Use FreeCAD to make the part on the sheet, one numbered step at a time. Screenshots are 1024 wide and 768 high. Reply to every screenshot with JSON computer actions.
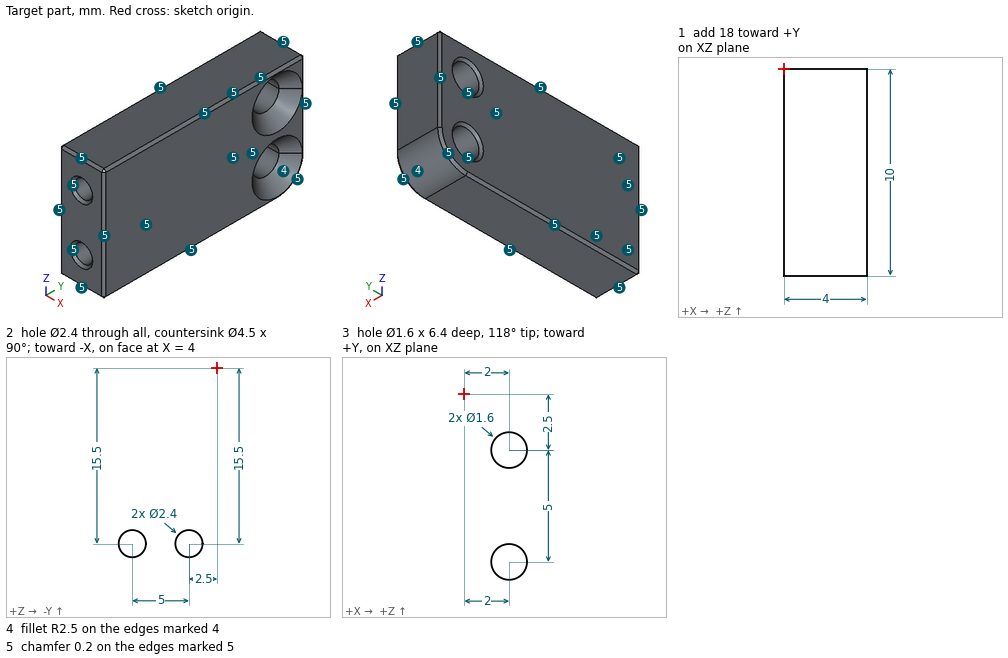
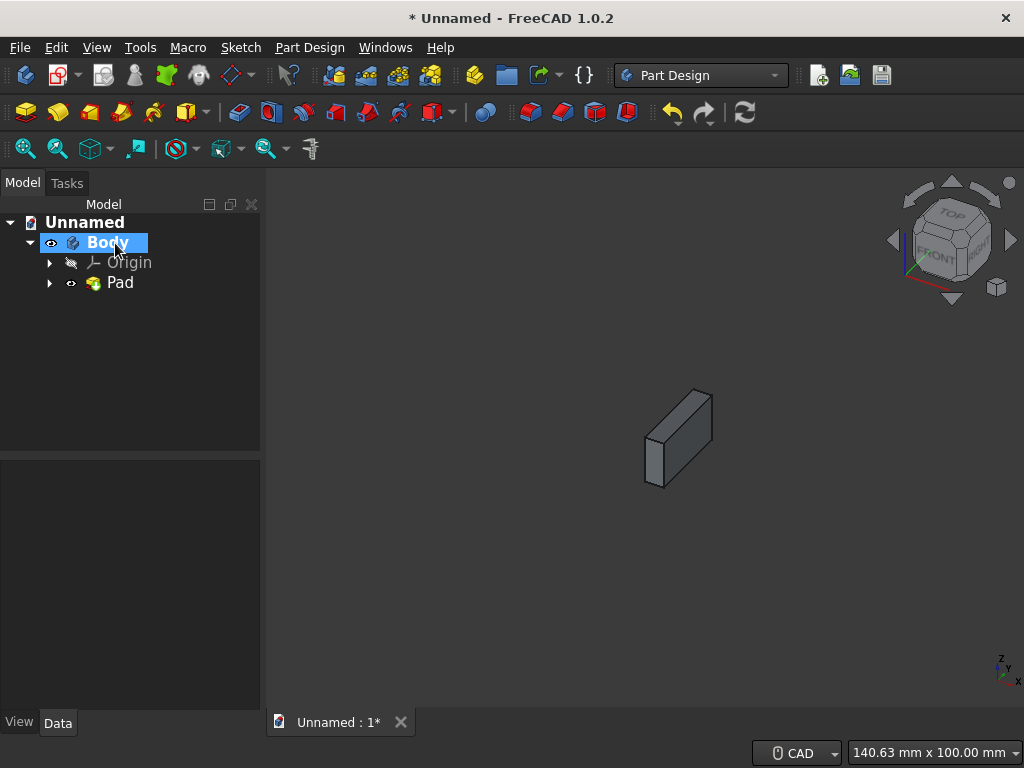
{"action": "left_click", "coordinate": [26, 150]}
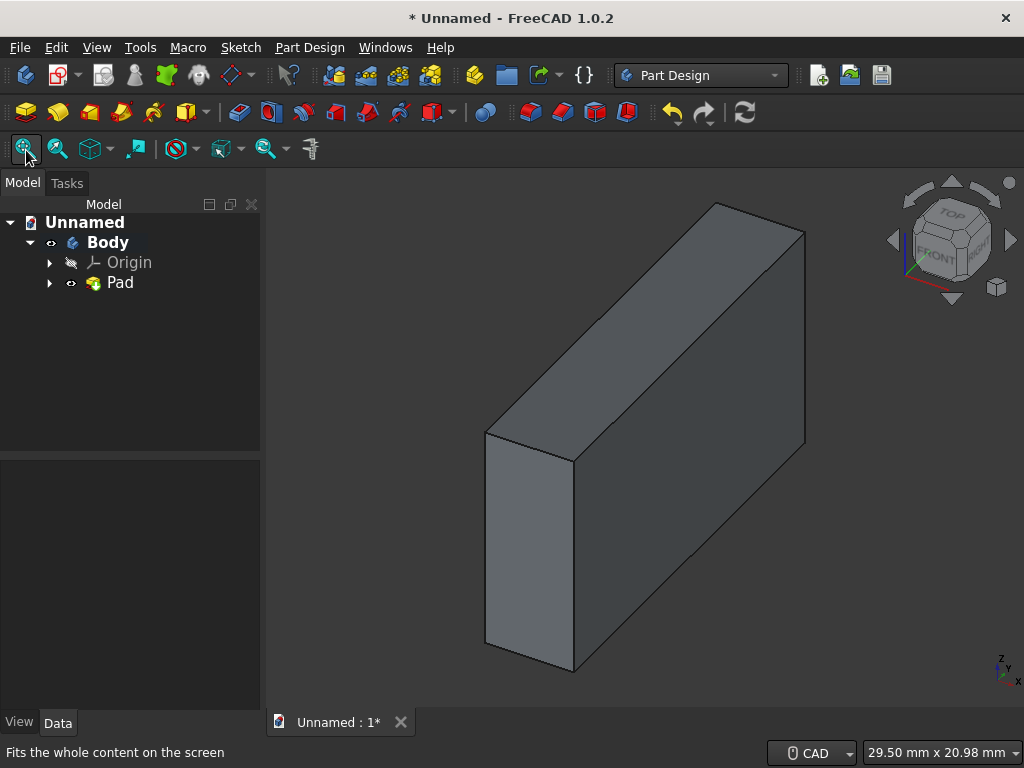
{"action": "left_click", "coordinate": [690, 451]}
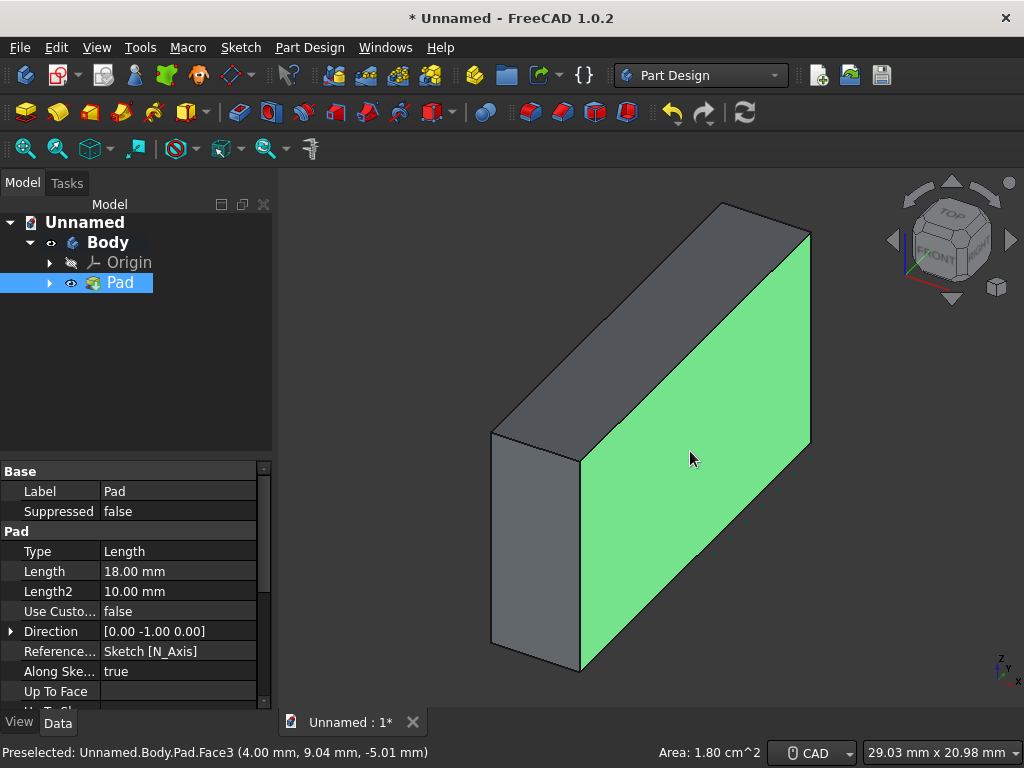
{"action": "left_click", "coordinate": [58, 76]}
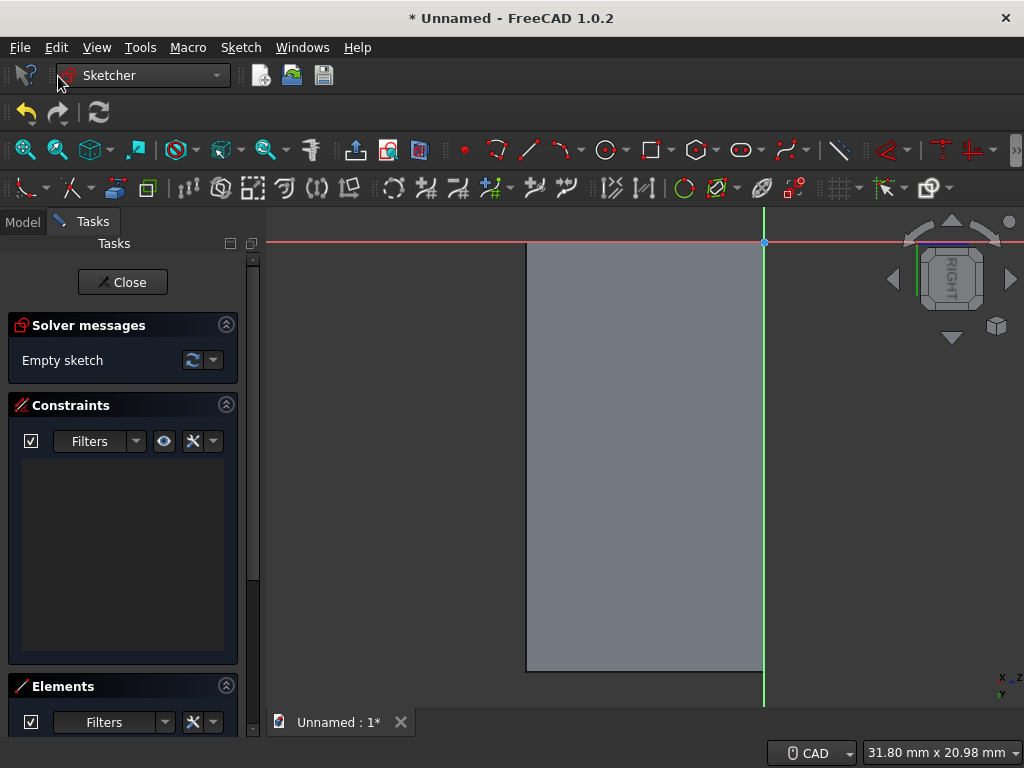
{"action": "scroll", "coordinate": [294, 527], "scroll_direction": "down", "scroll_amount": 1}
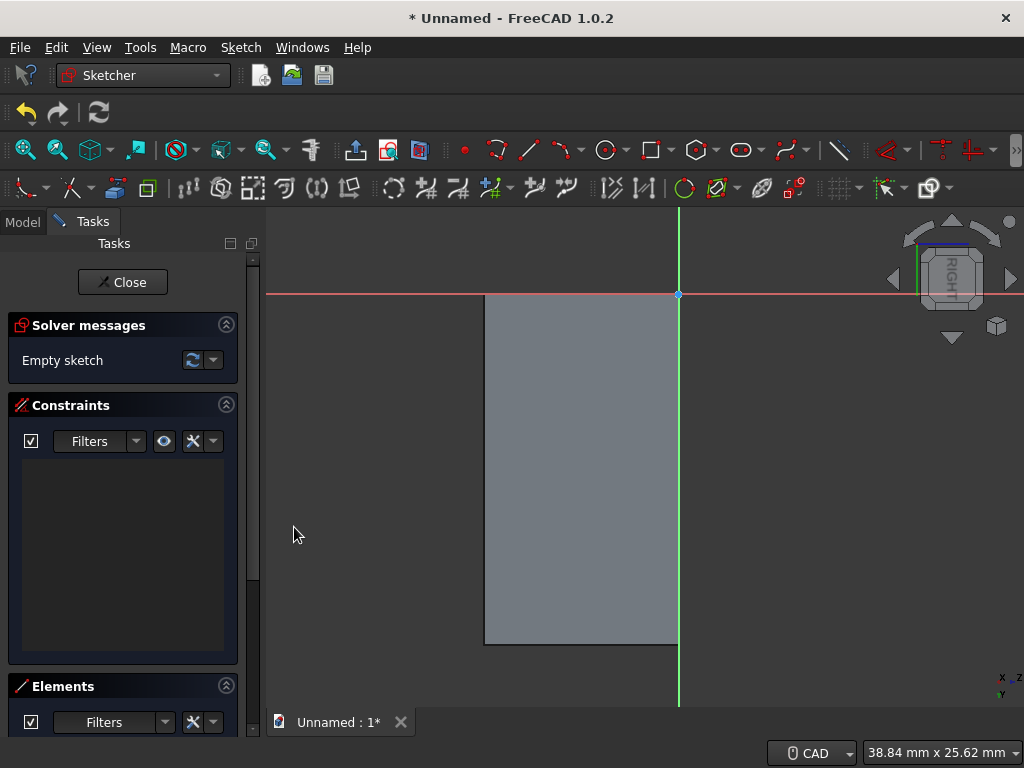
{"action": "key", "text": "g c"}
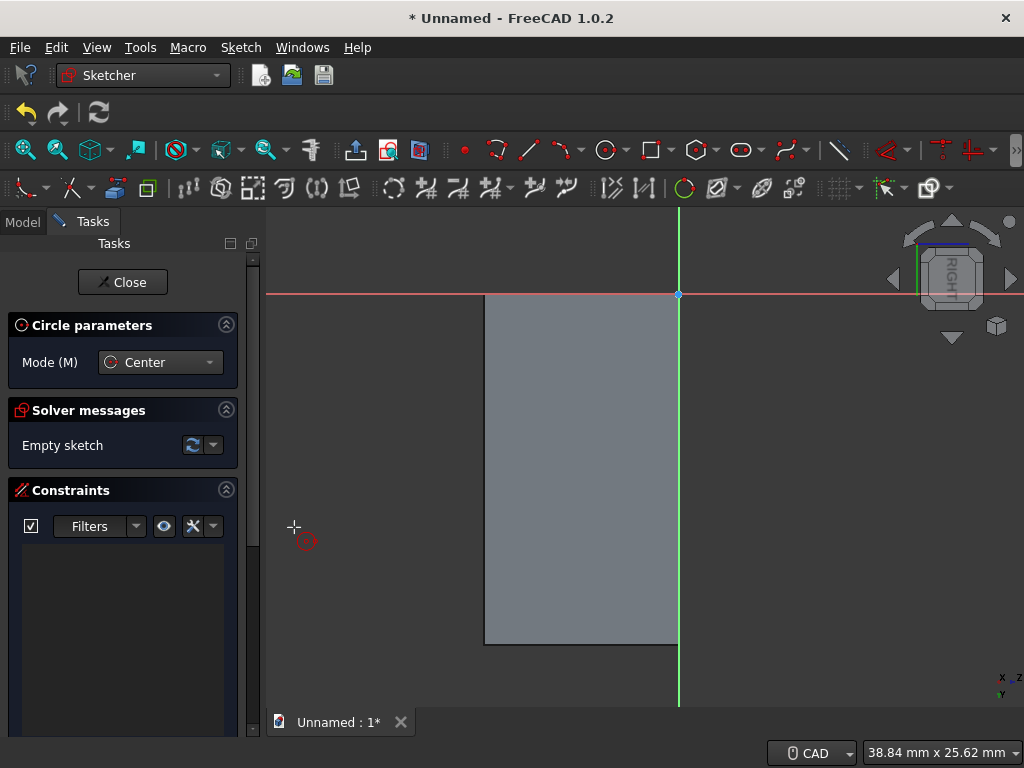
{"action": "left_click", "coordinate": [630, 597]}
{"action": "mouse_move", "coordinate": [647, 580]}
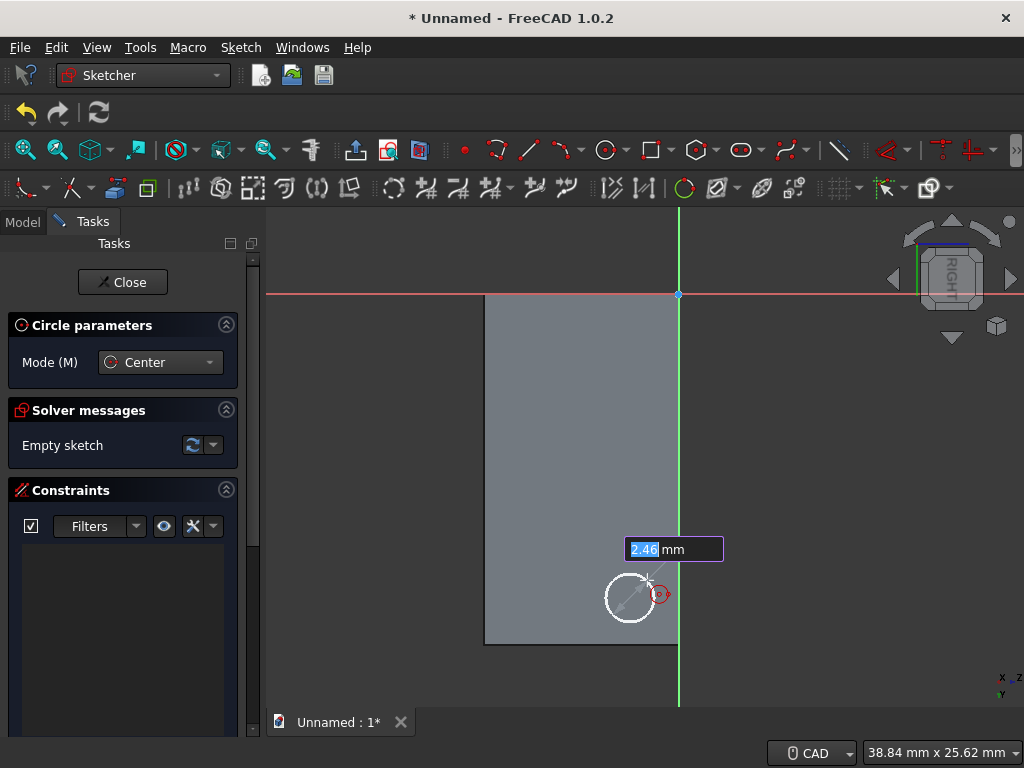
{"action": "type", "text": "2.4"}
{"action": "key", "text": "Return"}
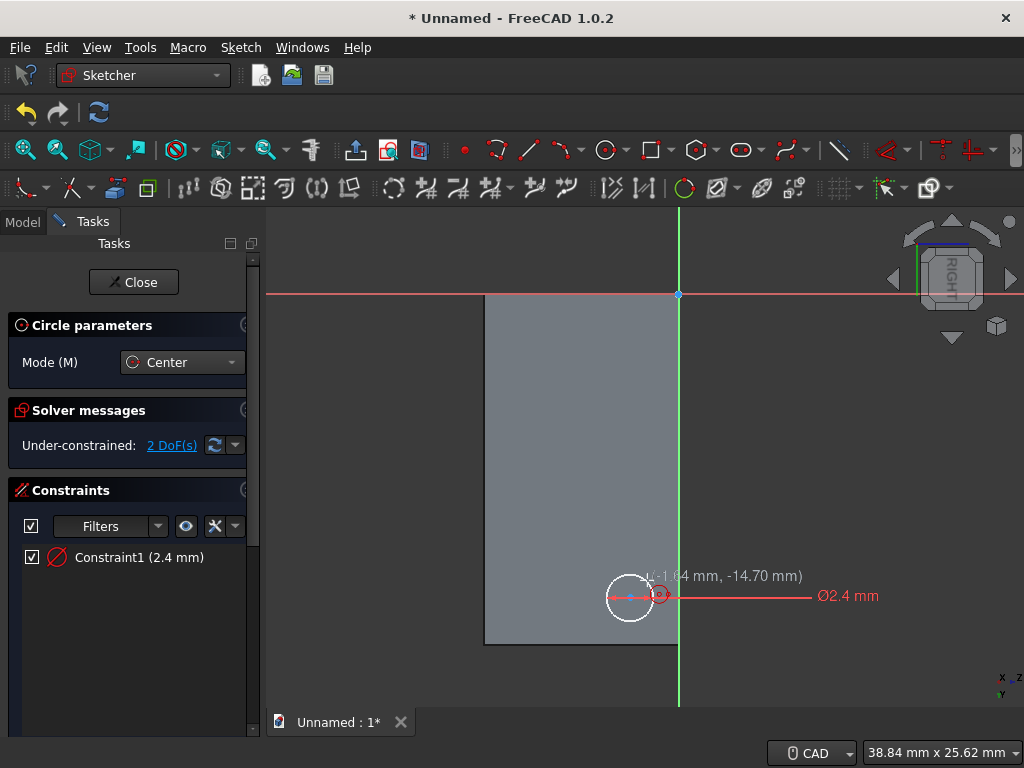
{"action": "left_click", "coordinate": [533, 597]}
{"action": "mouse_move", "coordinate": [549, 580]}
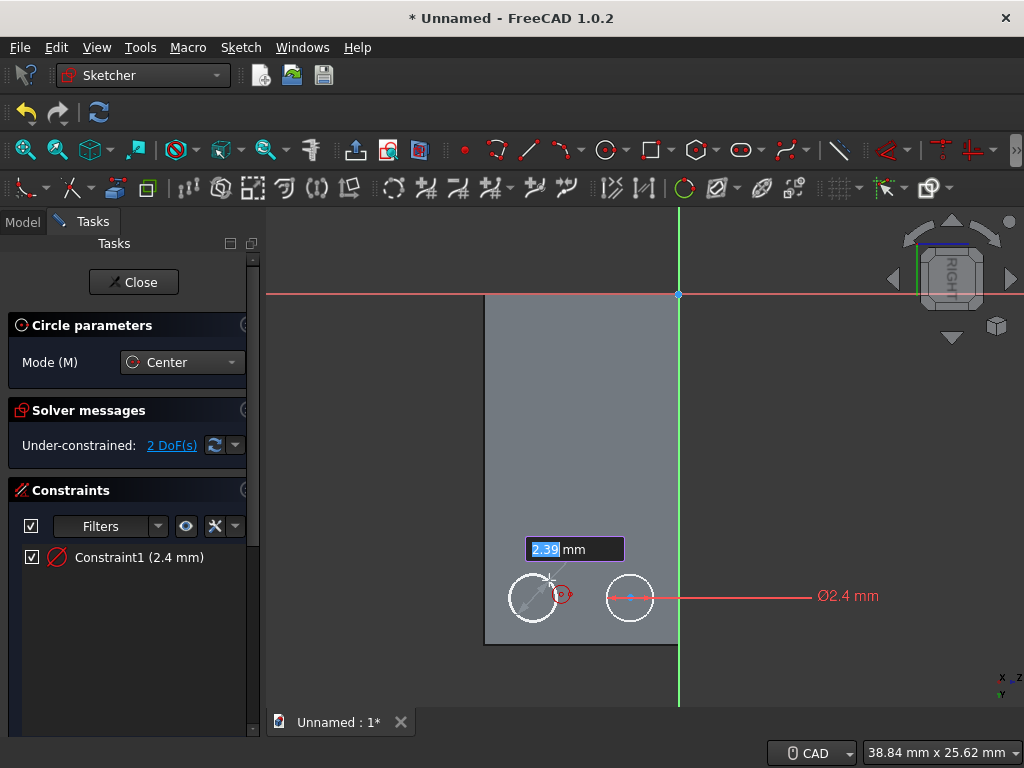
{"action": "type", "text": "2.4"}
{"action": "key", "text": "Return"}
{"action": "key", "text": "Escape"}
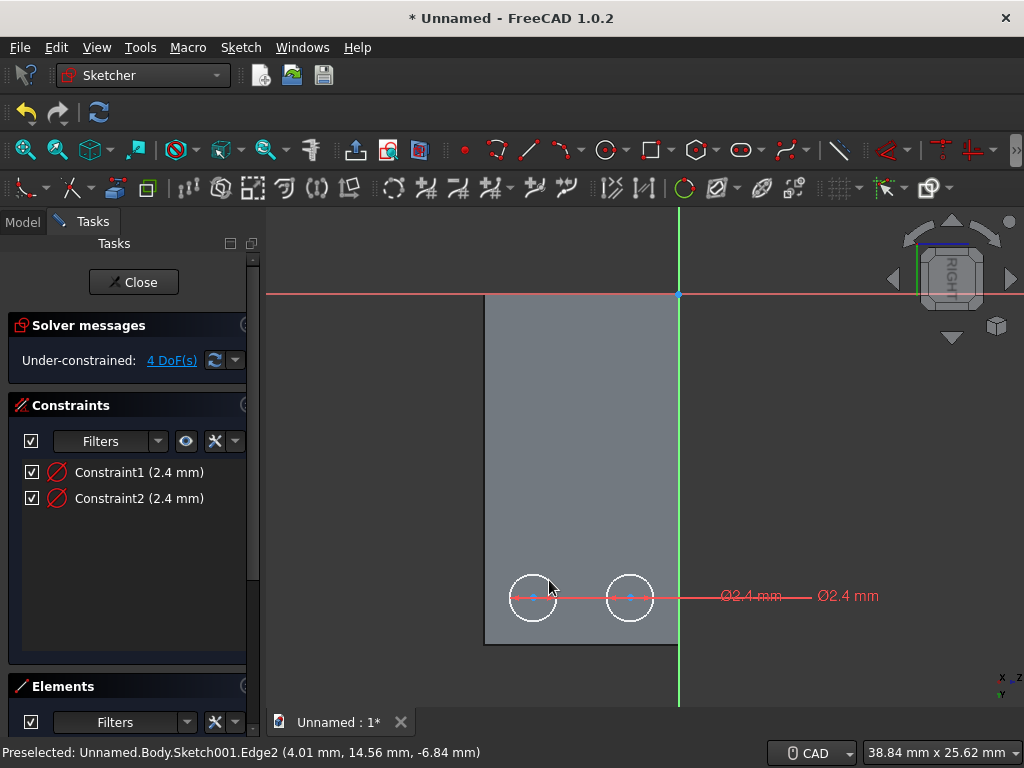
{"action": "key", "text": "d"}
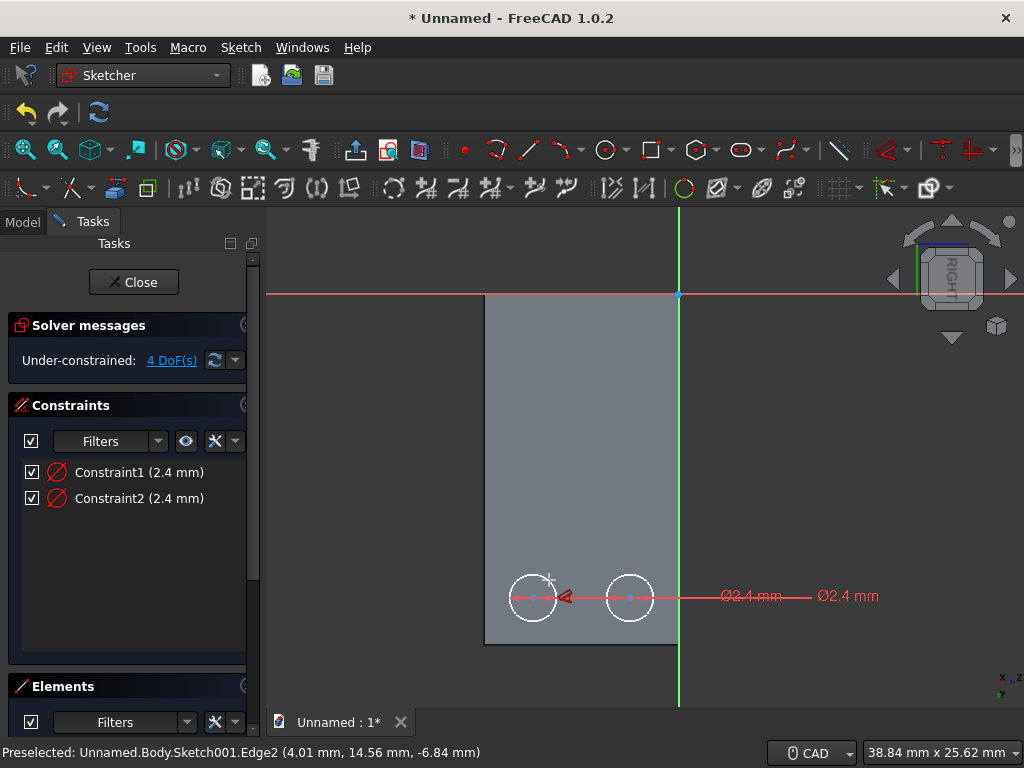
{"action": "left_click", "coordinate": [630, 598]}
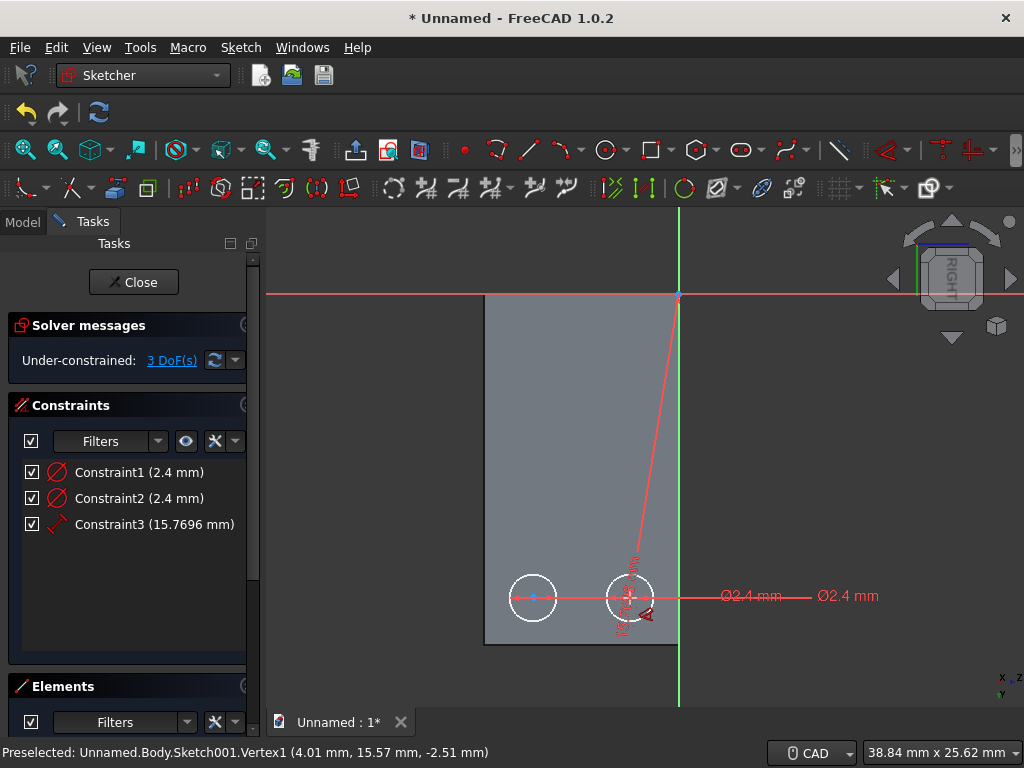
{"action": "left_click", "coordinate": [533, 598]}
{"action": "left_click", "coordinate": [581, 632]}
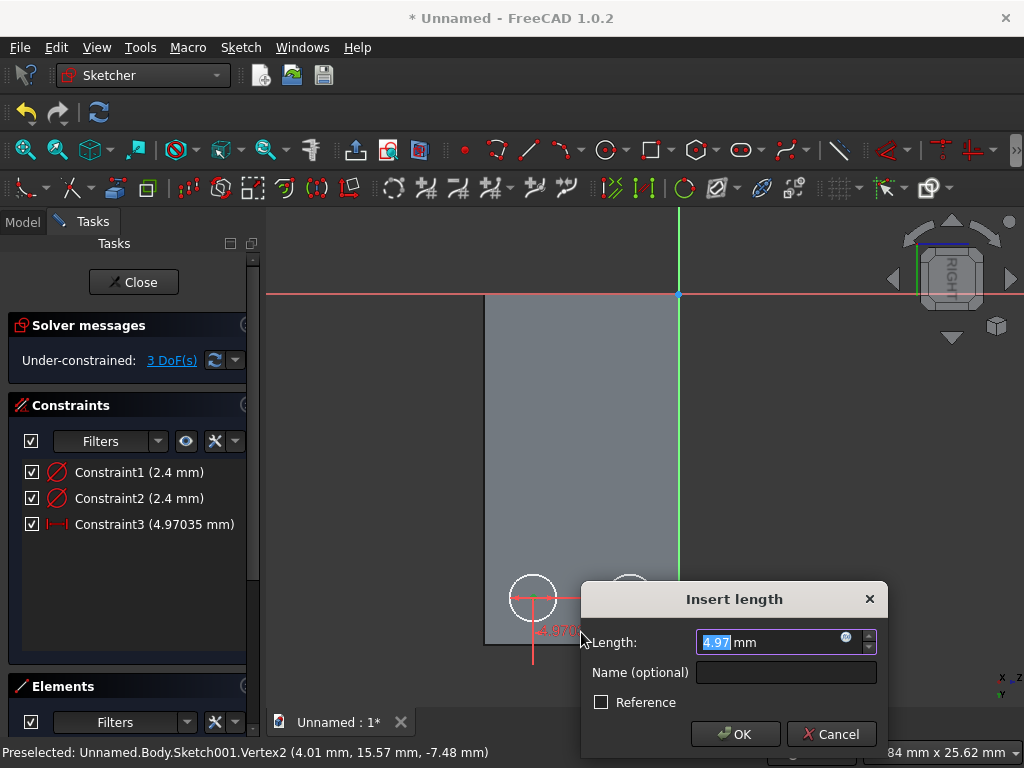
{"action": "type", "text": "5"}
{"action": "key", "text": "Return"}